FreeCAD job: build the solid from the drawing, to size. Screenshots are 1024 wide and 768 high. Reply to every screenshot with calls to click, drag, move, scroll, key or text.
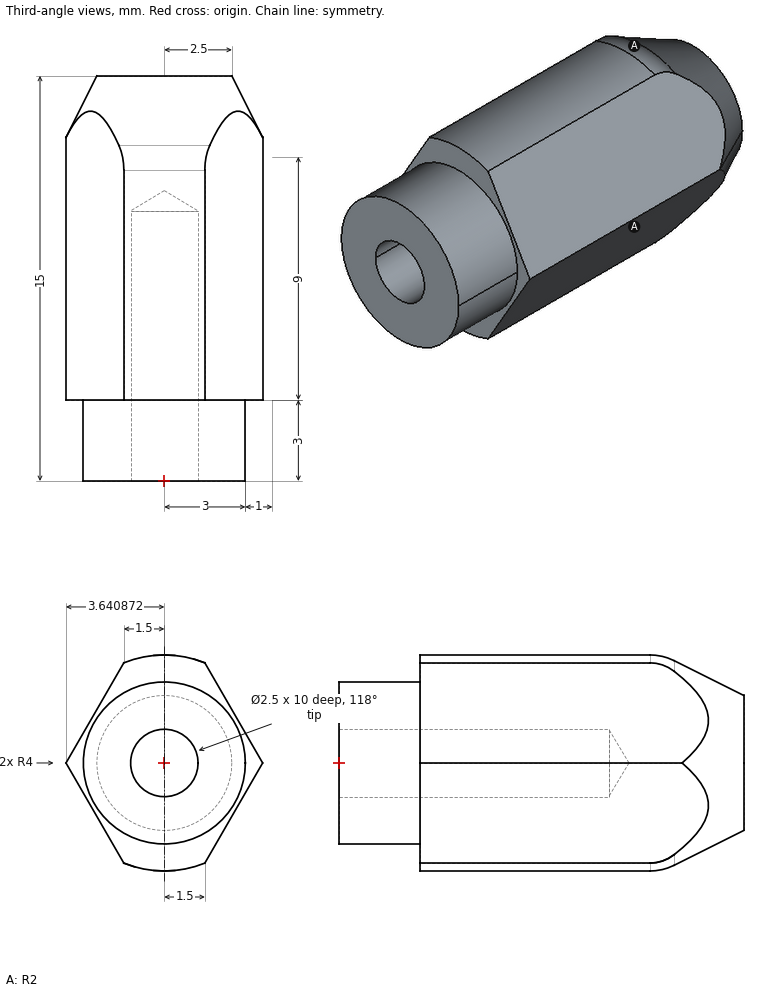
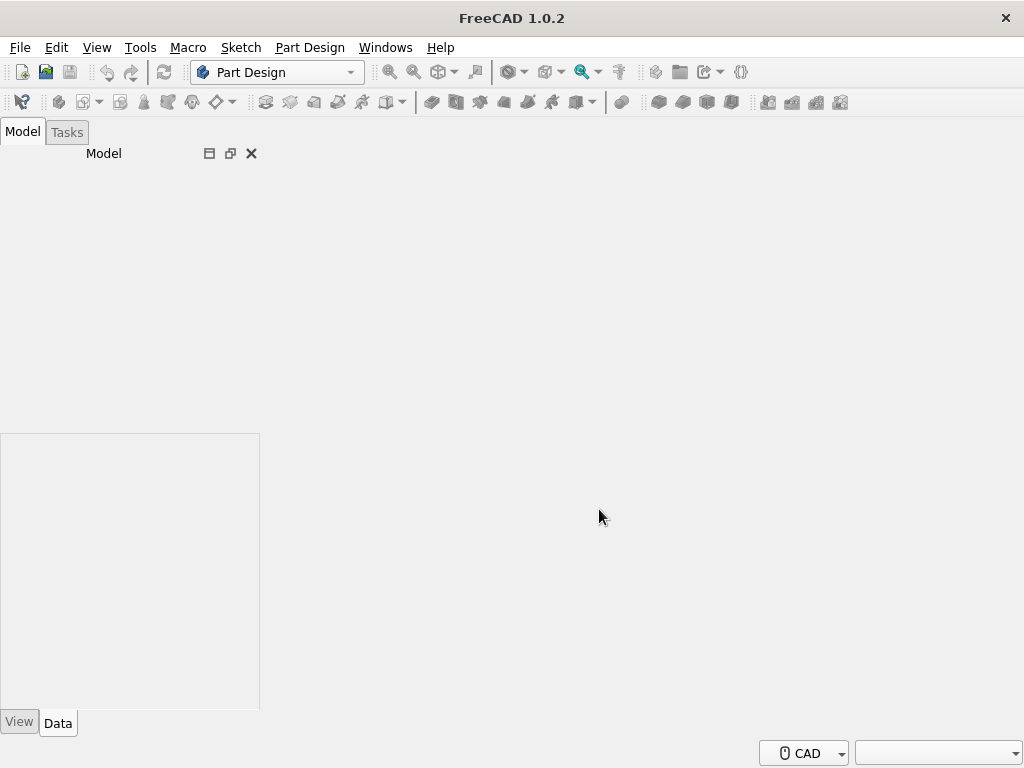
click(22, 72)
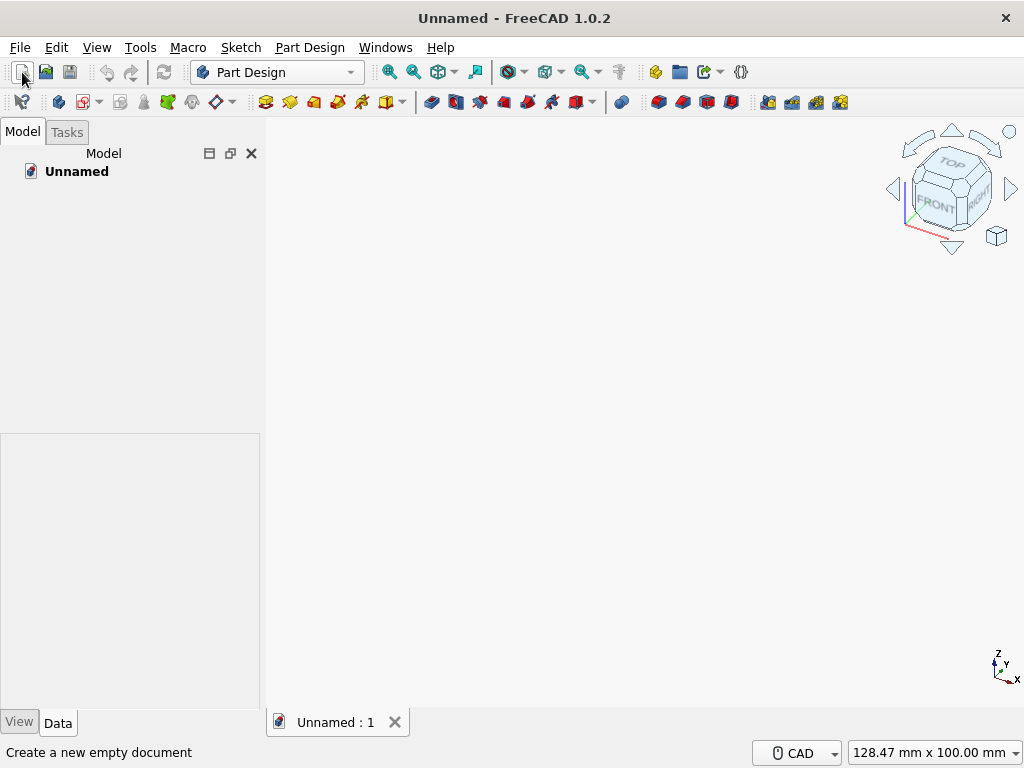
click(84, 102)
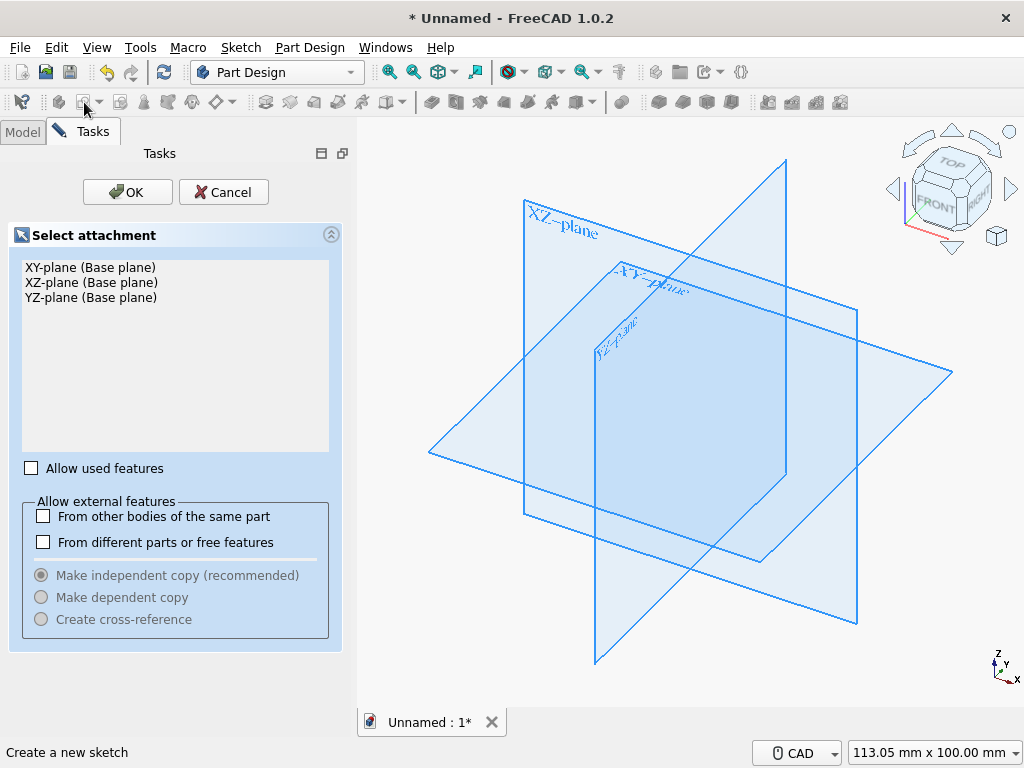
click(82, 268)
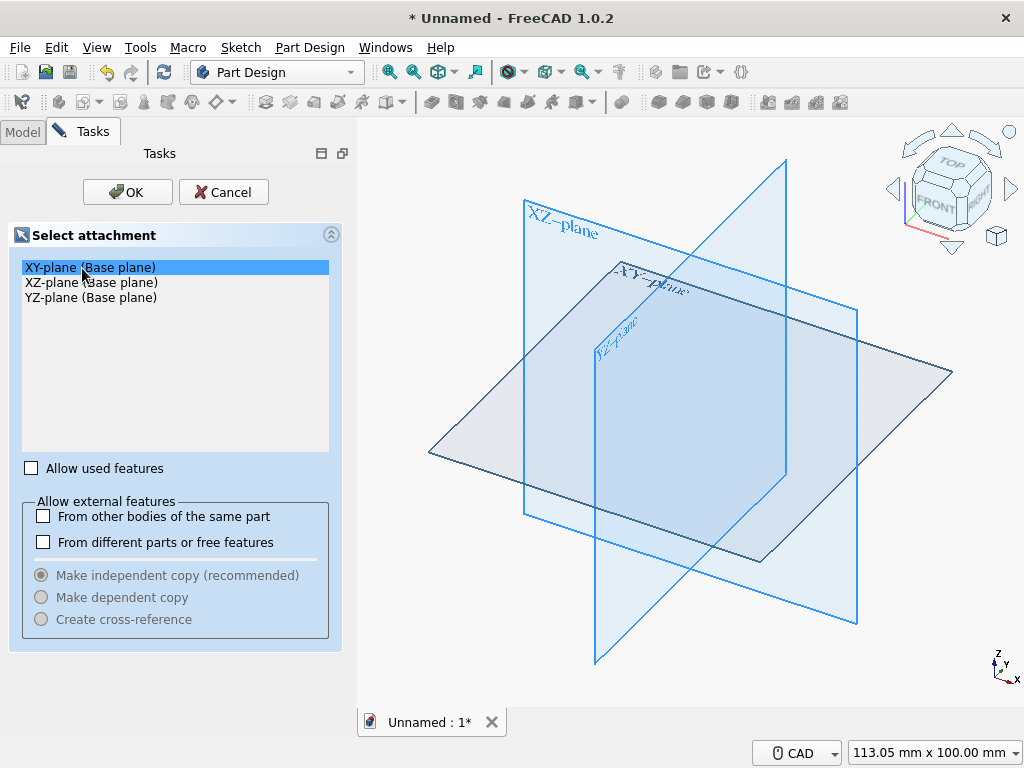
click(128, 192)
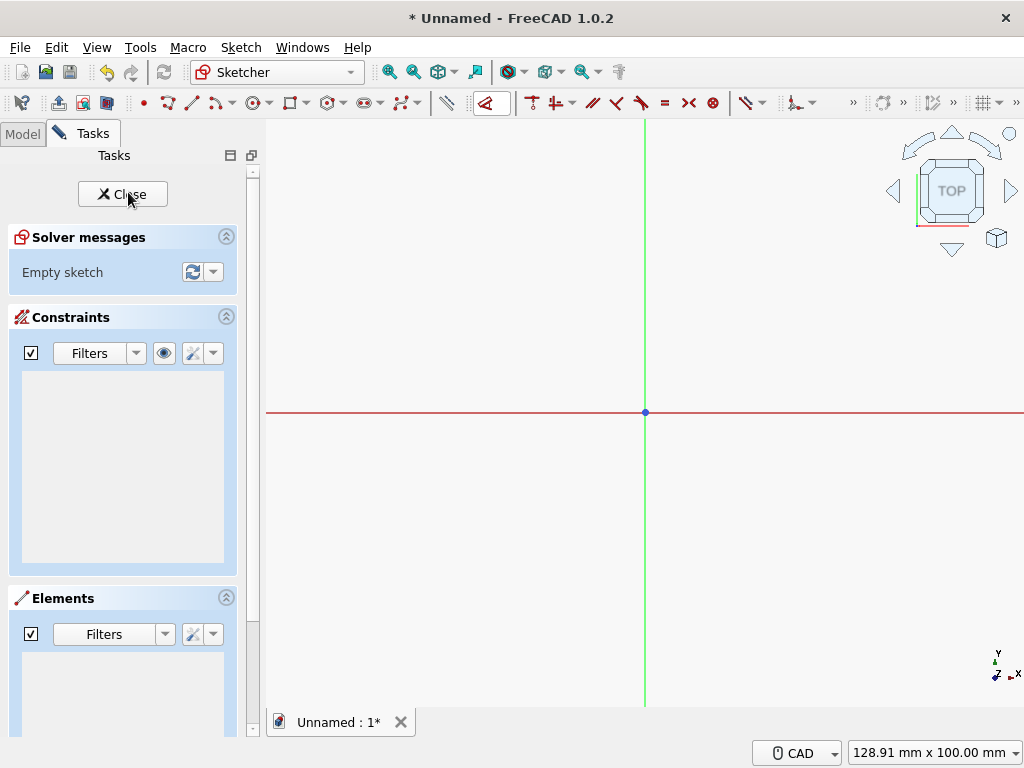
scroll(683, 354, up, 7)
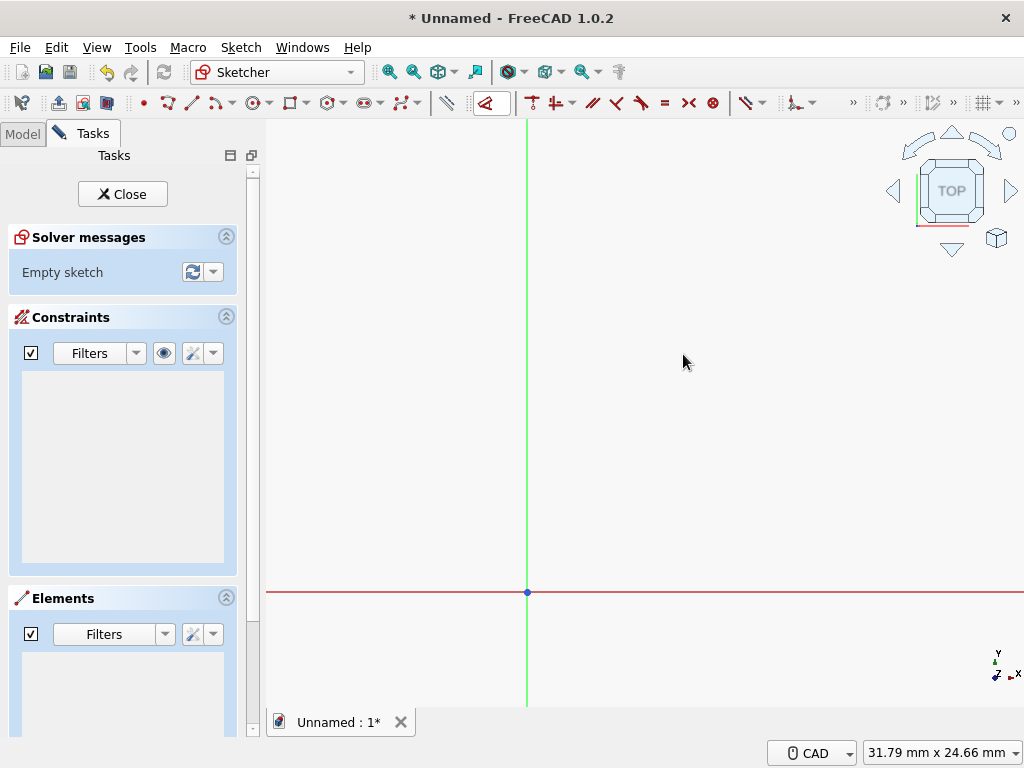
click(168, 104)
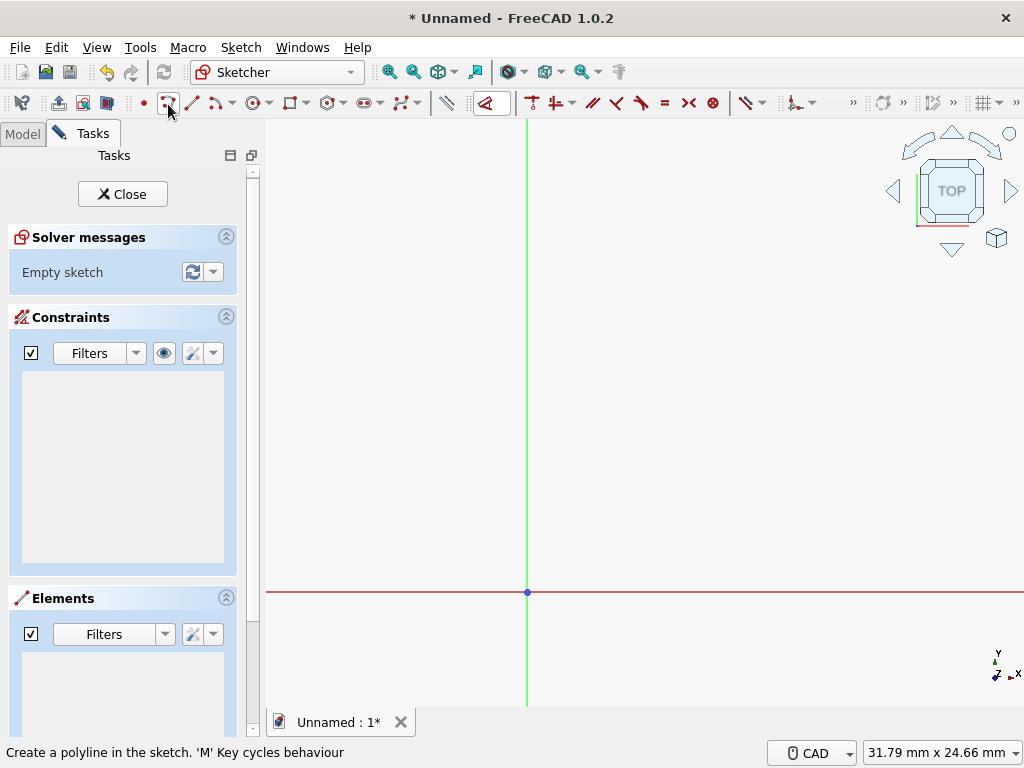
click(527, 592)
click(599, 583)
click(599, 520)
click(623, 520)
click(623, 306)
click(587, 234)
click(536, 234)
click(527, 592)
key(Escape)
key(Escape)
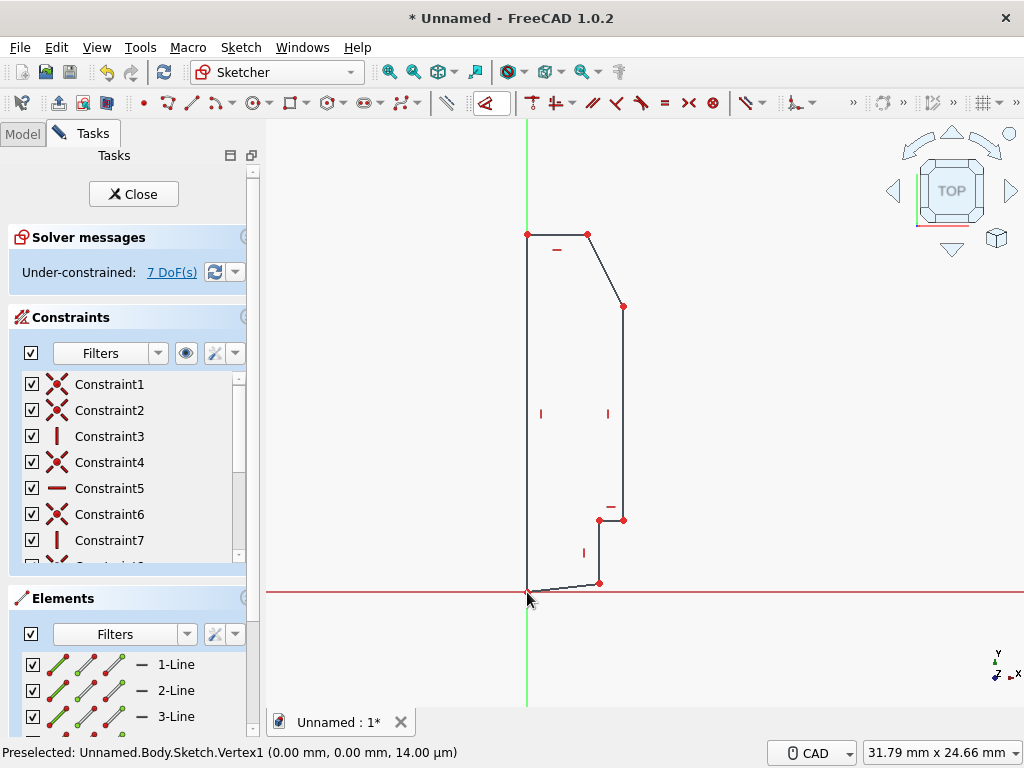
click(549, 590)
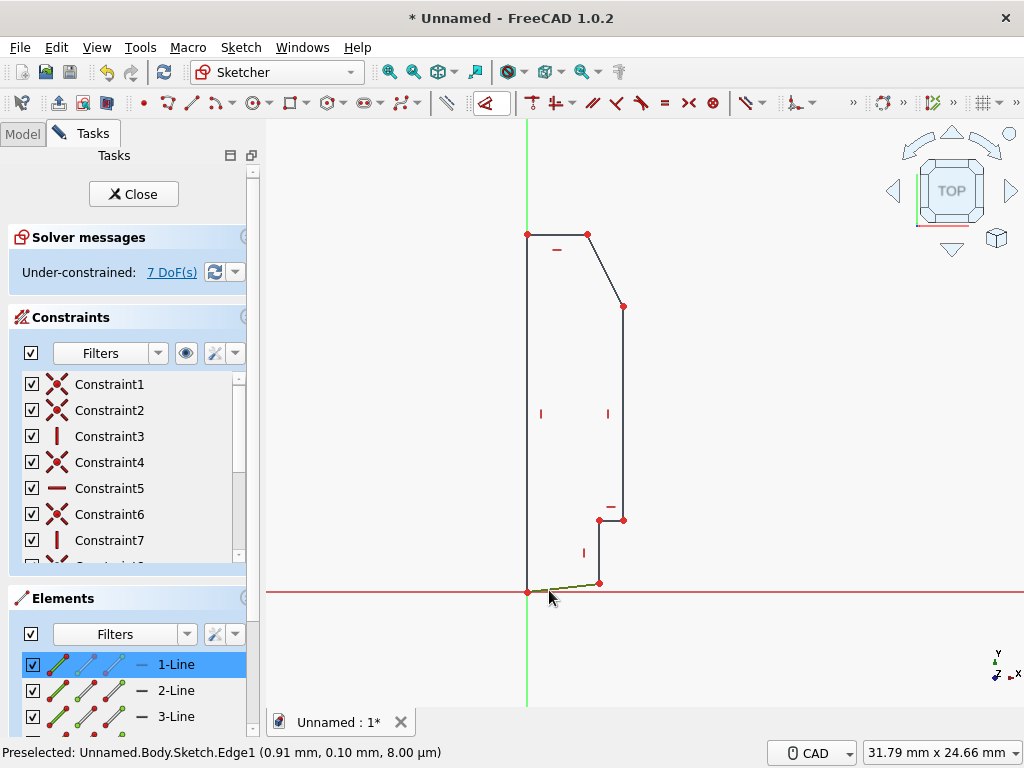
key(h)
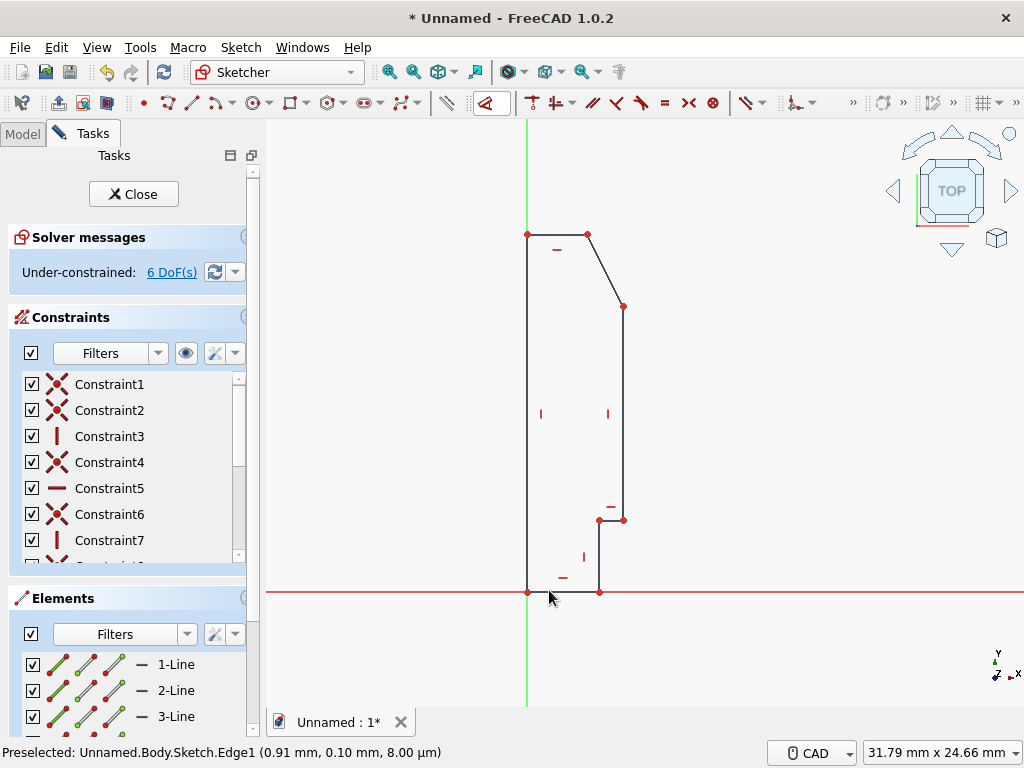
click(486, 104)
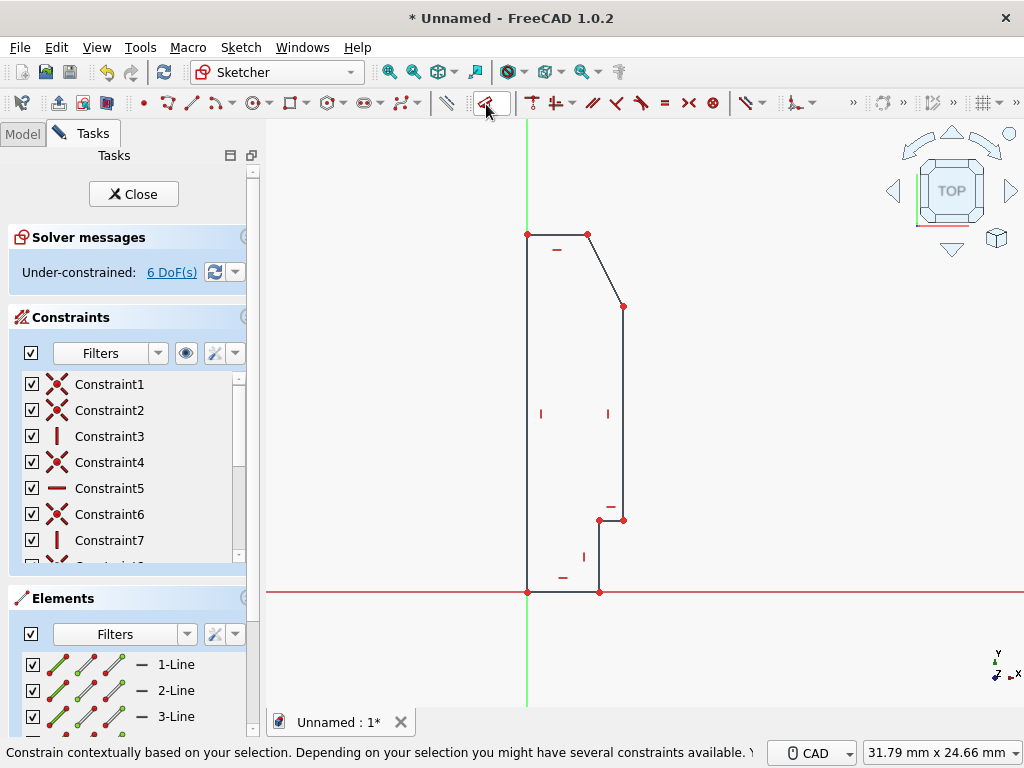
click(549, 592)
click(563, 626)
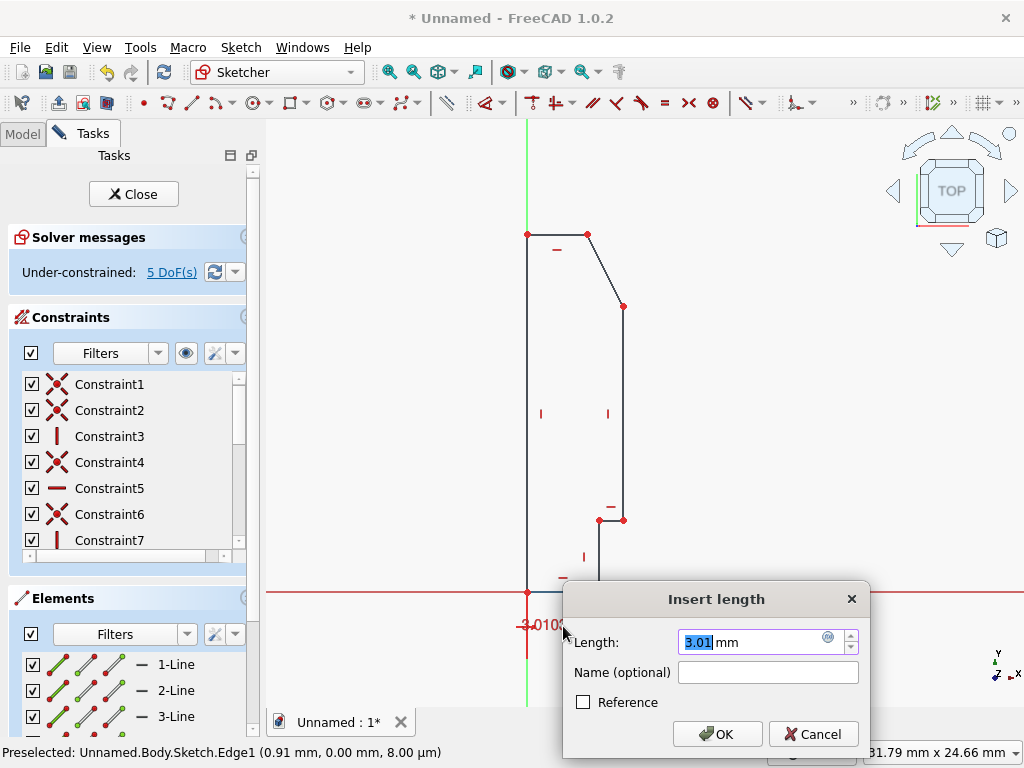
text(3)
key(Return)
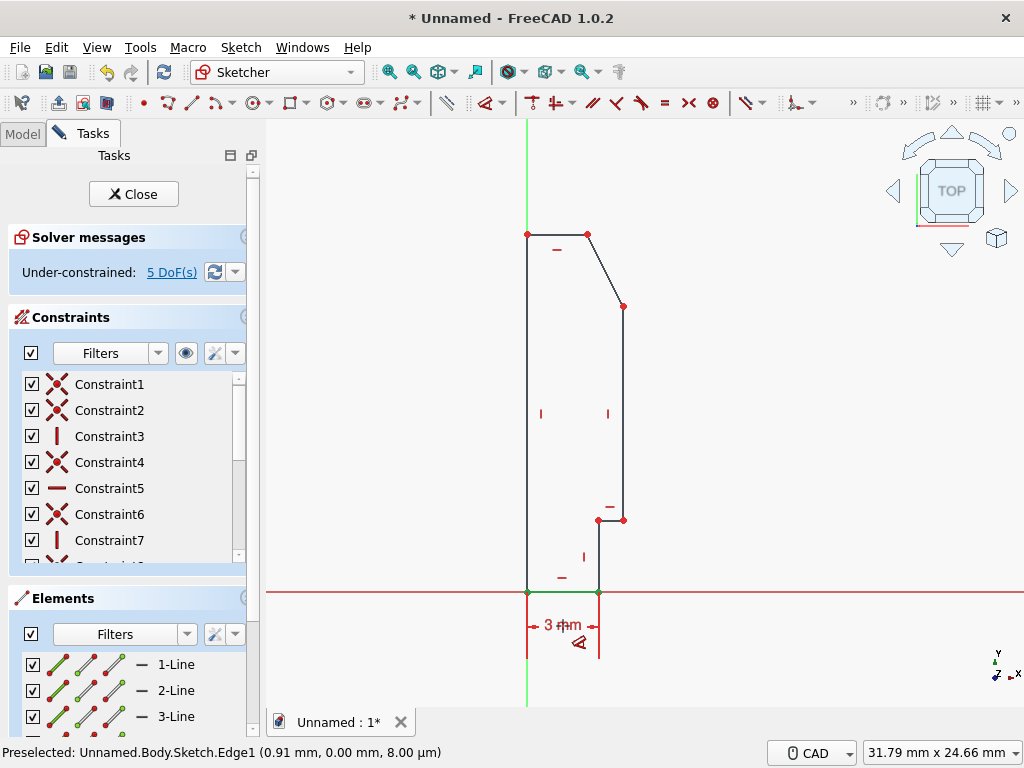
click(599, 571)
click(633, 557)